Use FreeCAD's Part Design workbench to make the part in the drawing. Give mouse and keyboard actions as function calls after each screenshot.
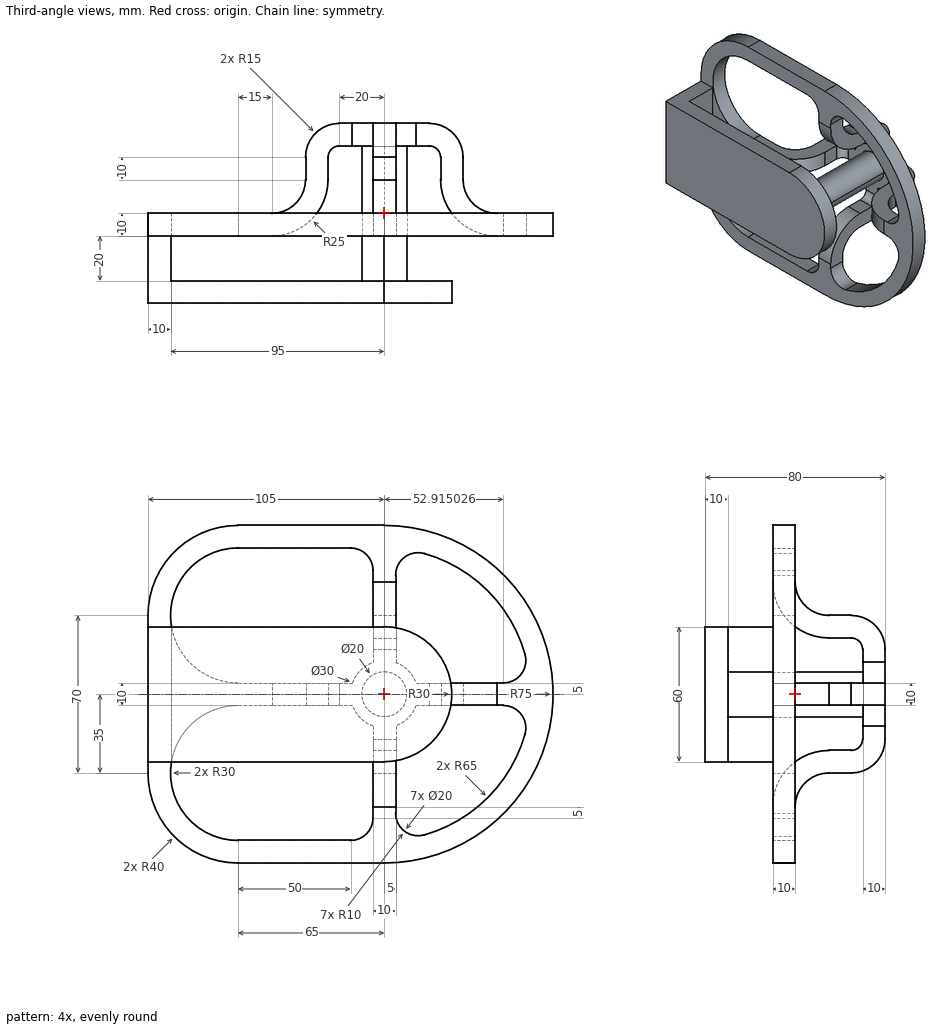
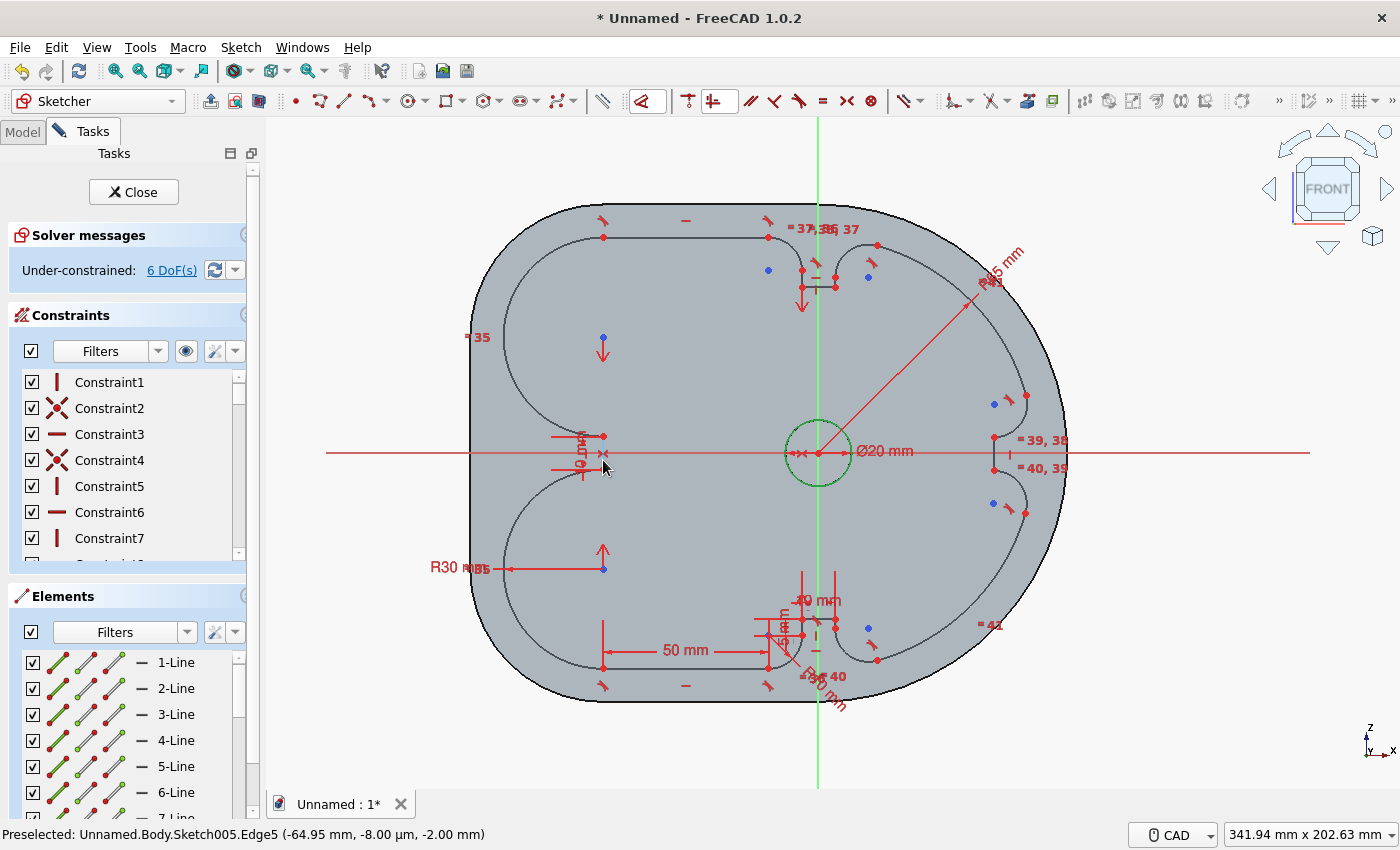
scroll(812, 287, up, 4)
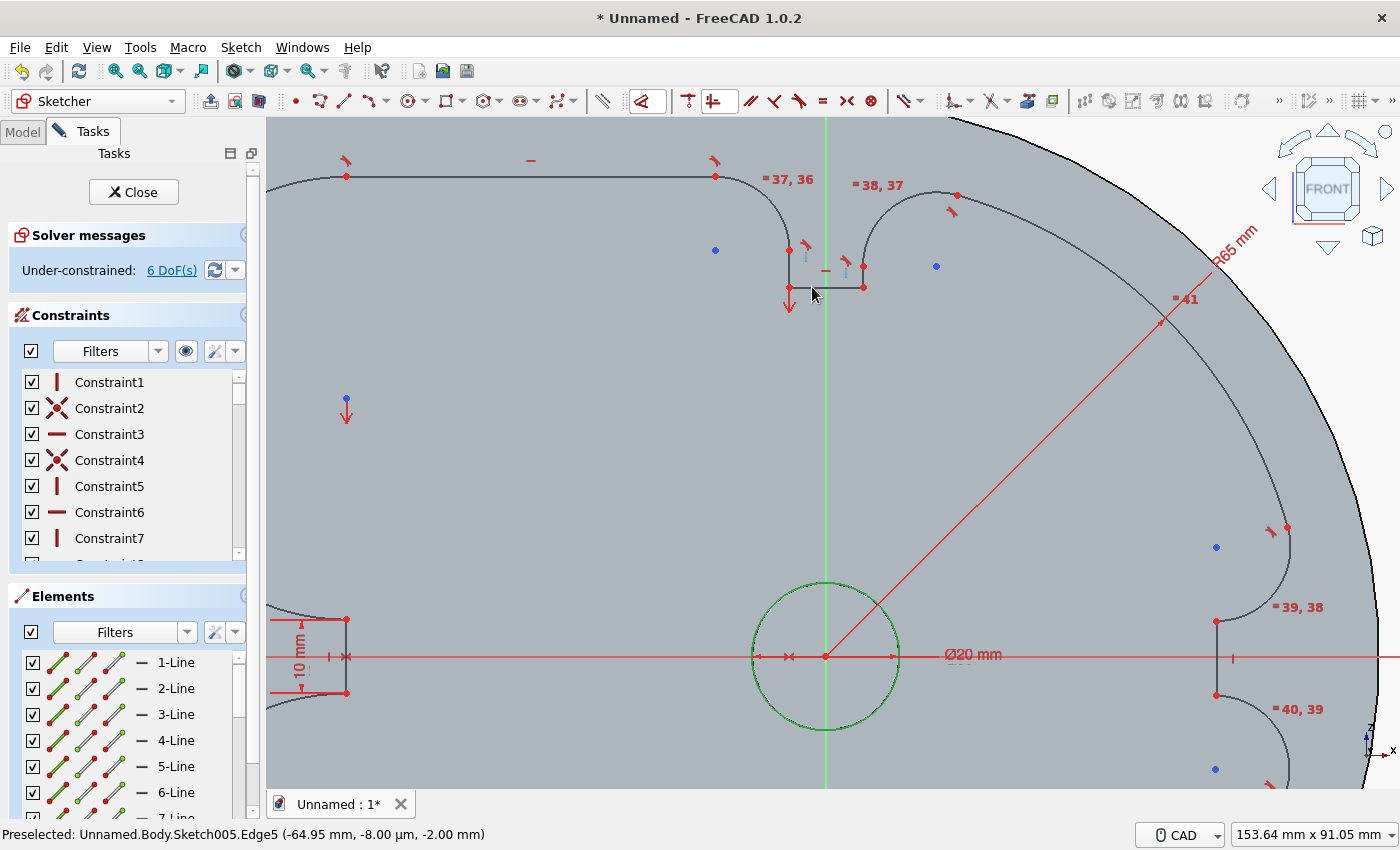
click(811, 288)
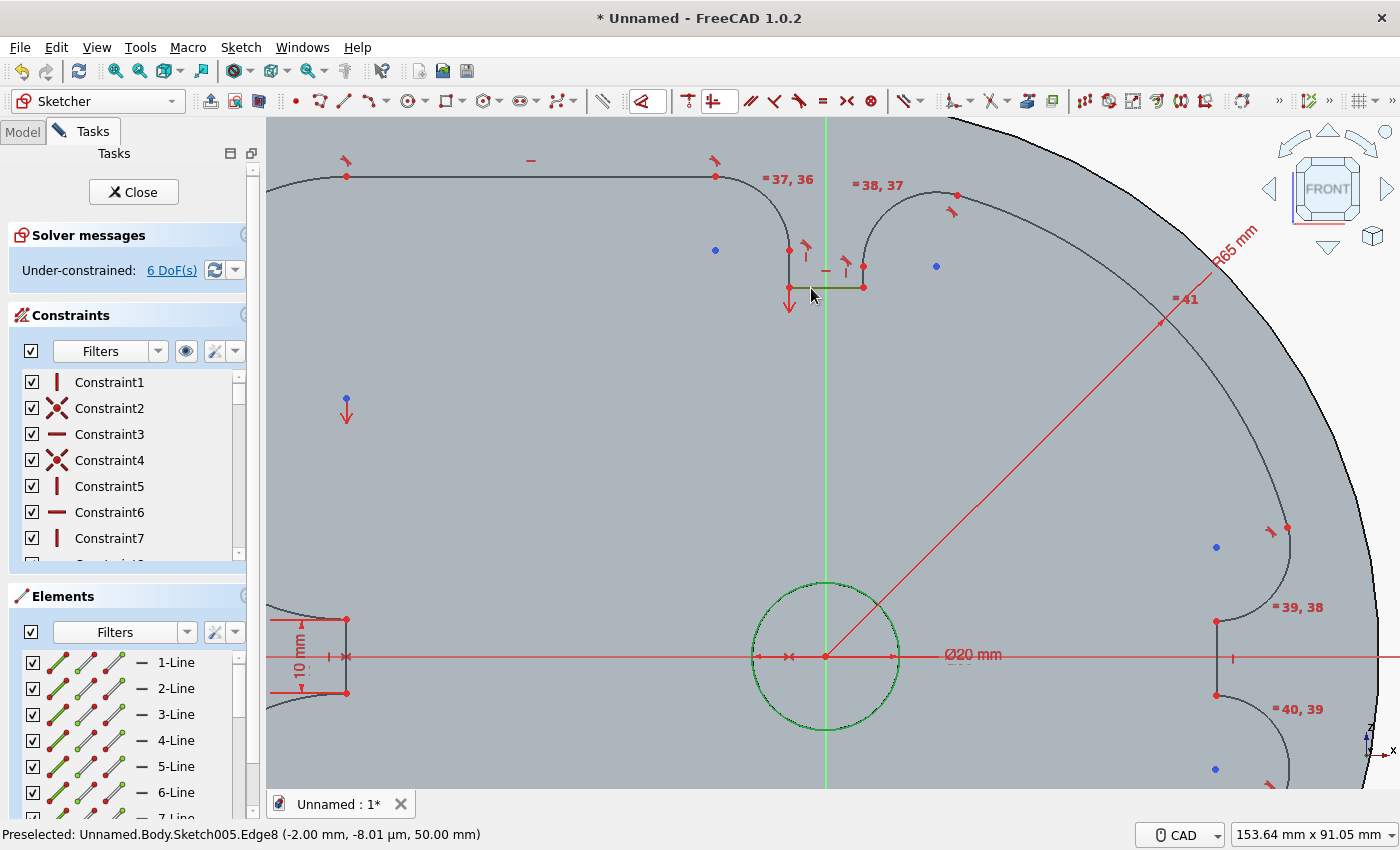
click(660, 102)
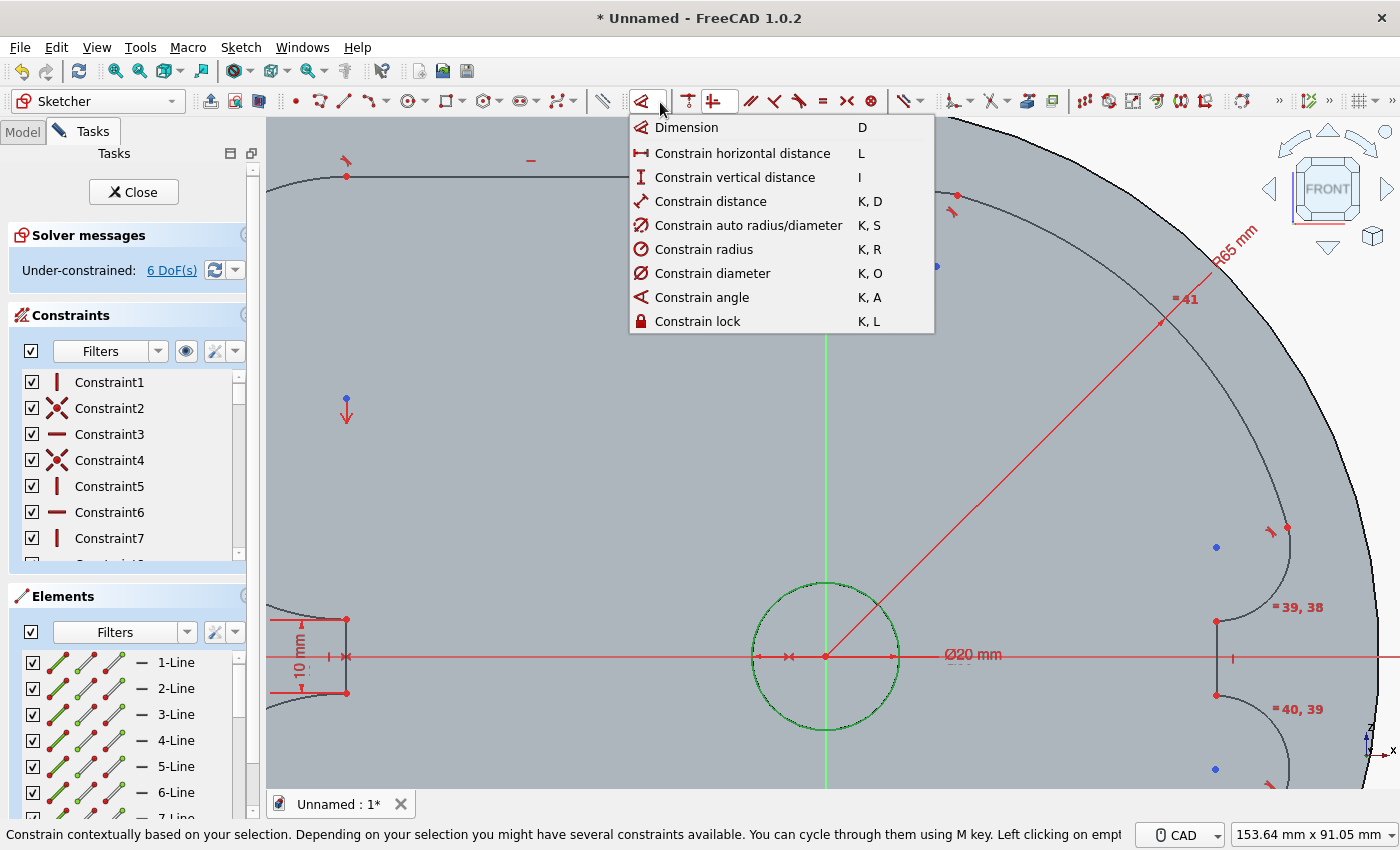
click(782, 153)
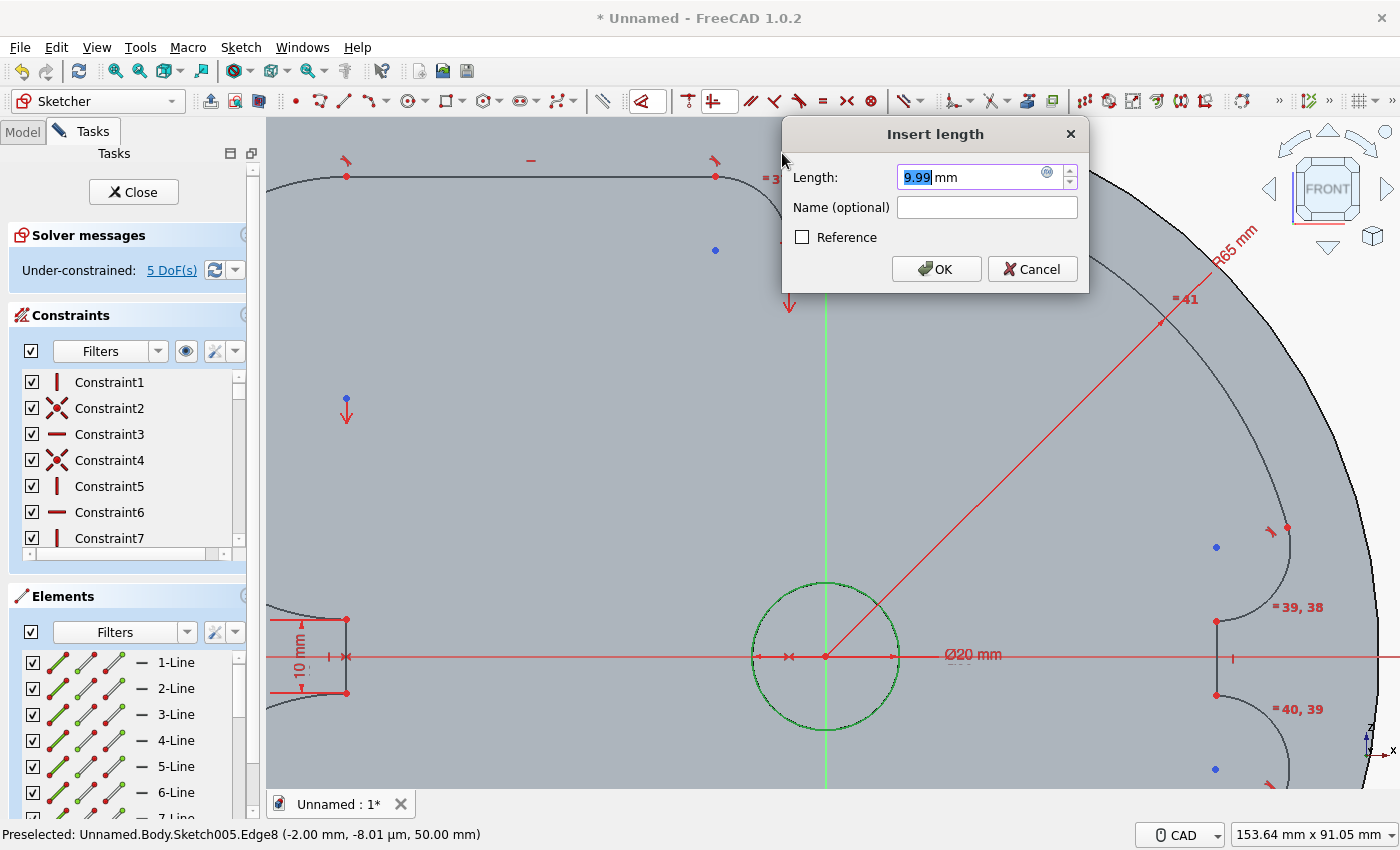
text(10)
key(Return)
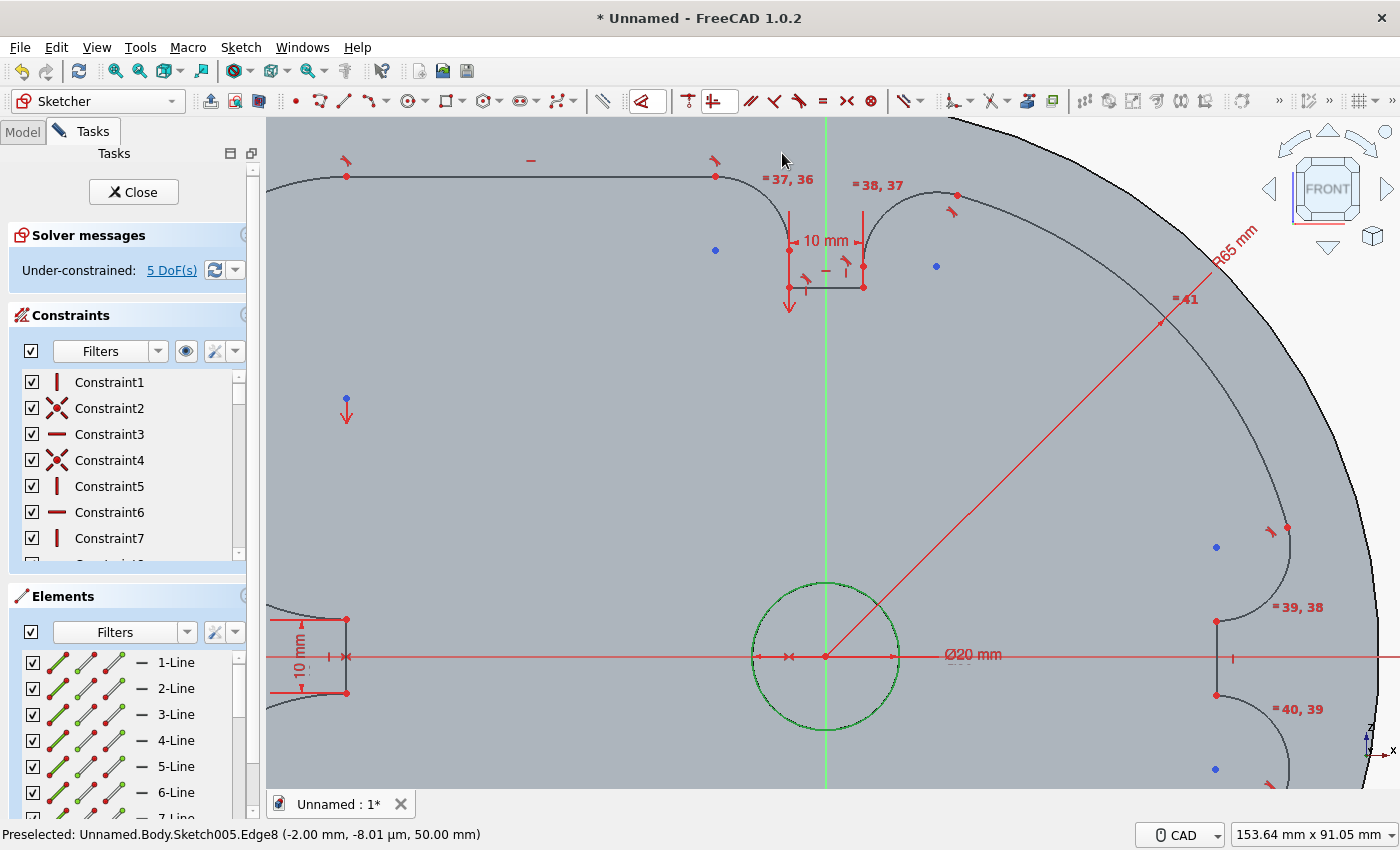
click(1217, 643)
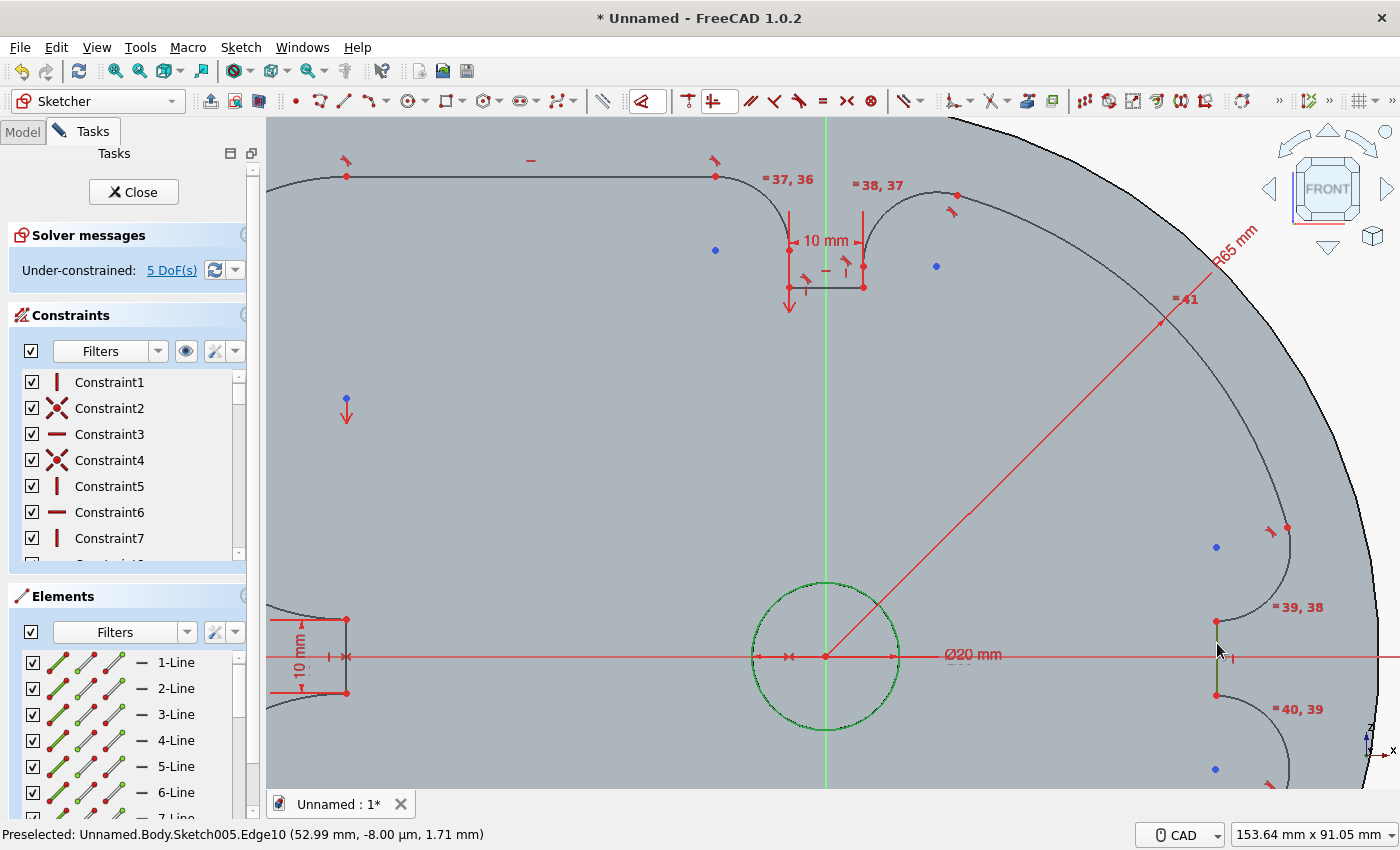
click(660, 102)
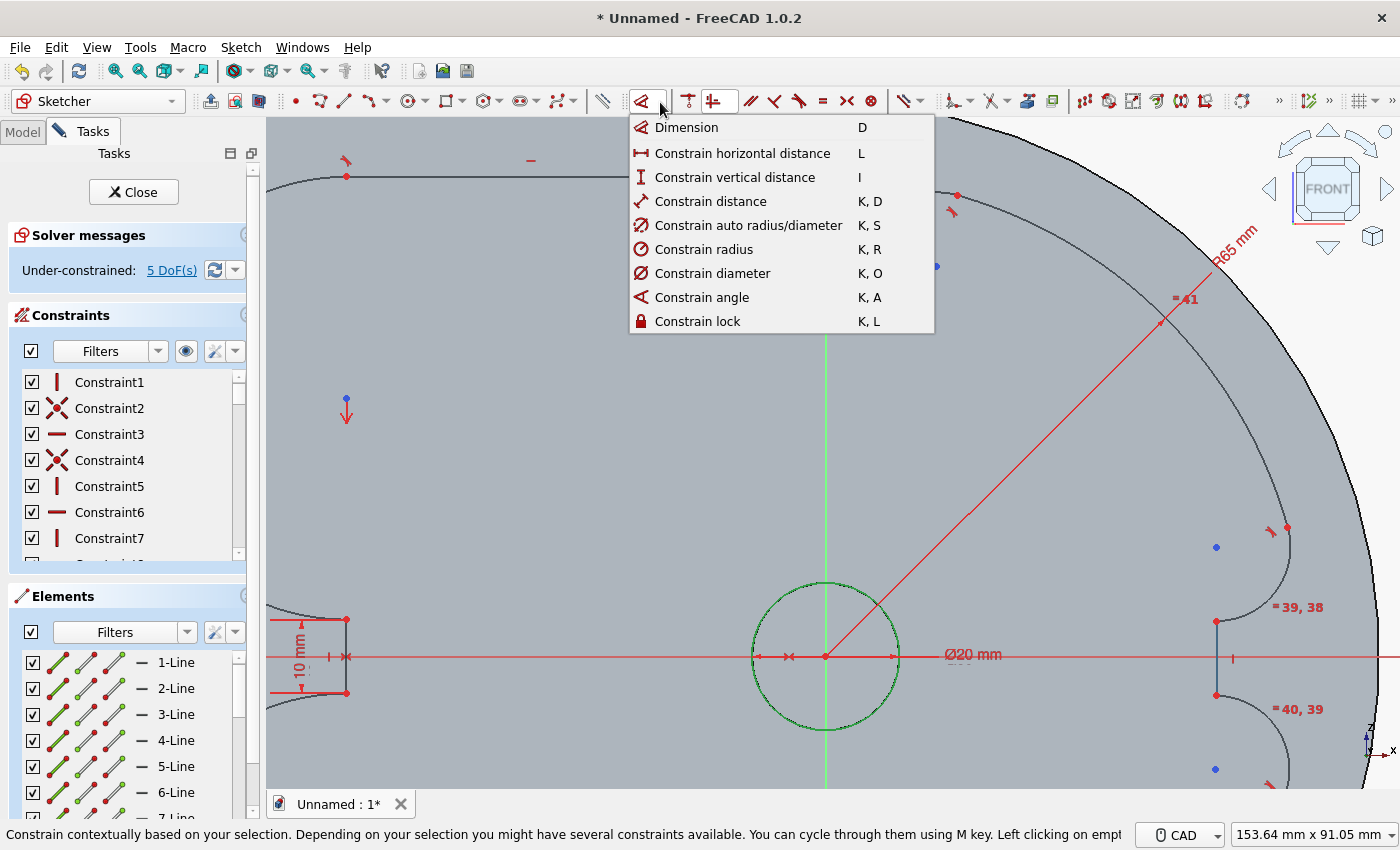
click(782, 177)